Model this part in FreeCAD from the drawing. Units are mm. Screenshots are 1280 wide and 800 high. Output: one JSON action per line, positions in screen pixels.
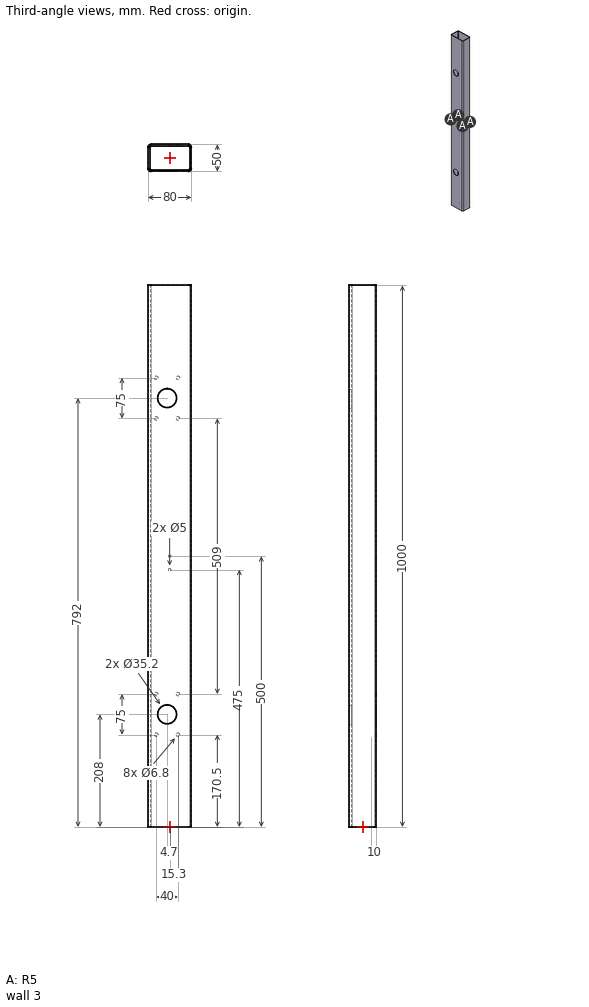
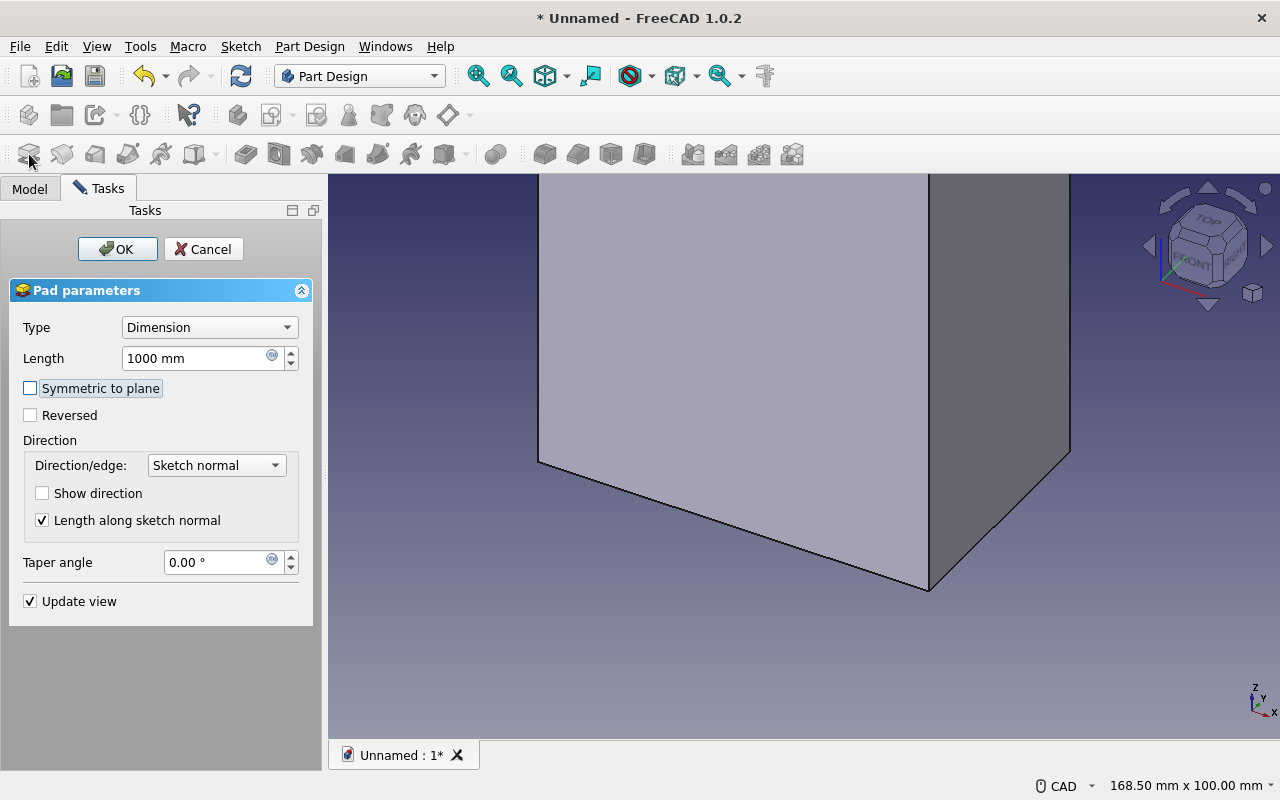
{"action": "left_click", "coordinate": [118, 249]}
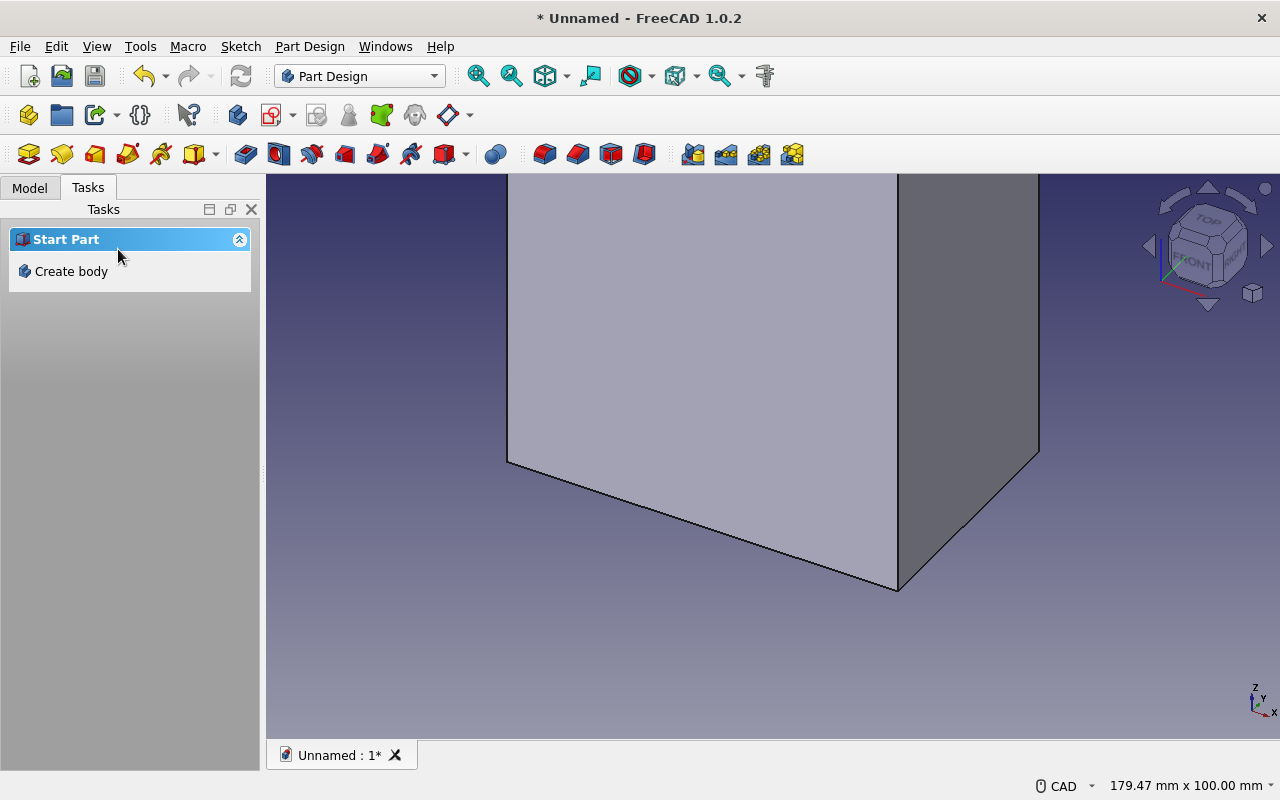
{"action": "left_click", "coordinate": [479, 76]}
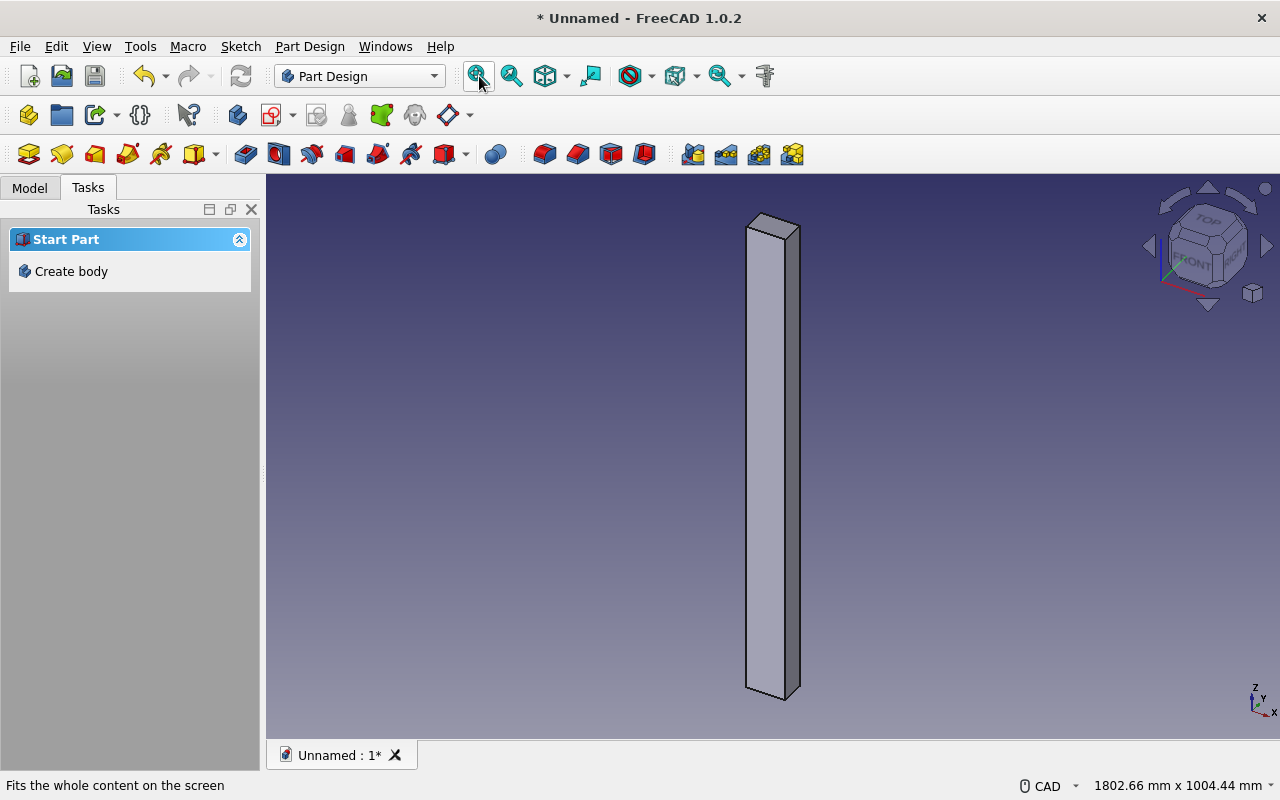
{"action": "left_click", "coordinate": [785, 469]}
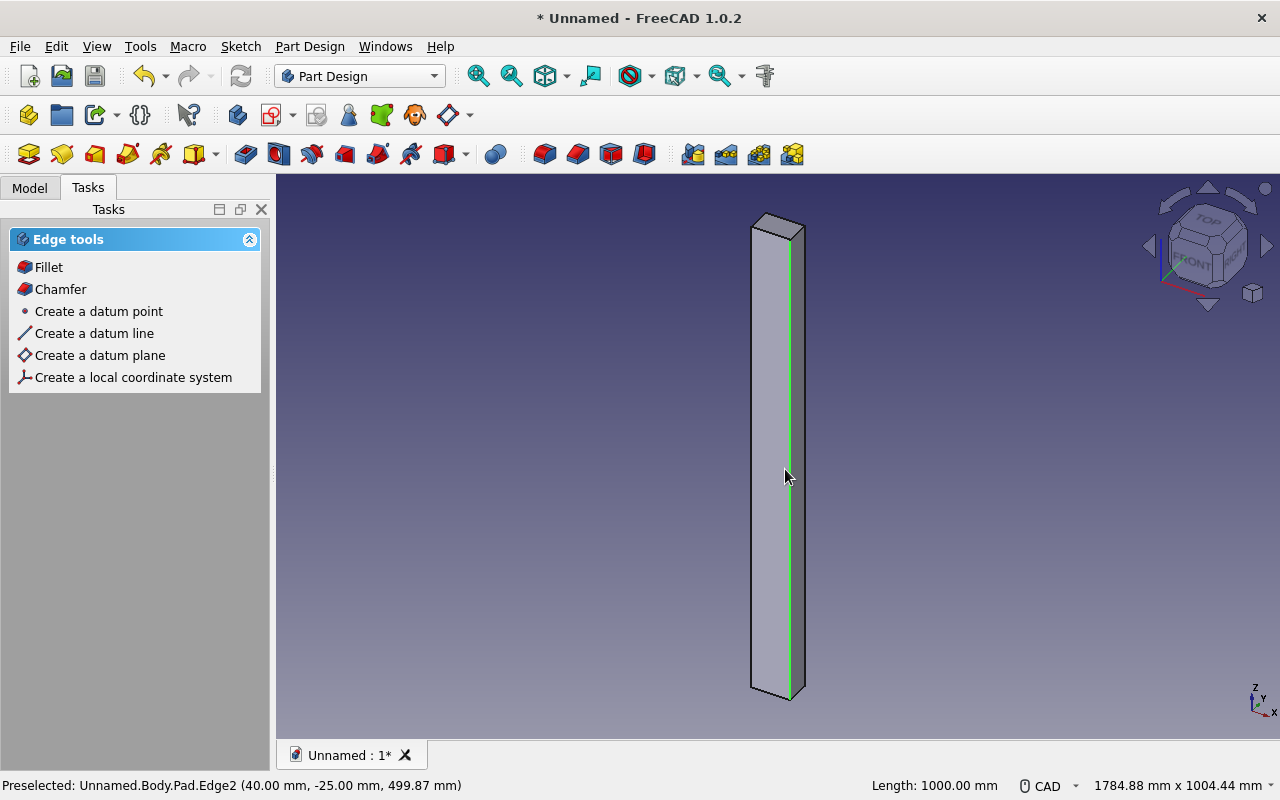
{"action": "key", "text": "0"}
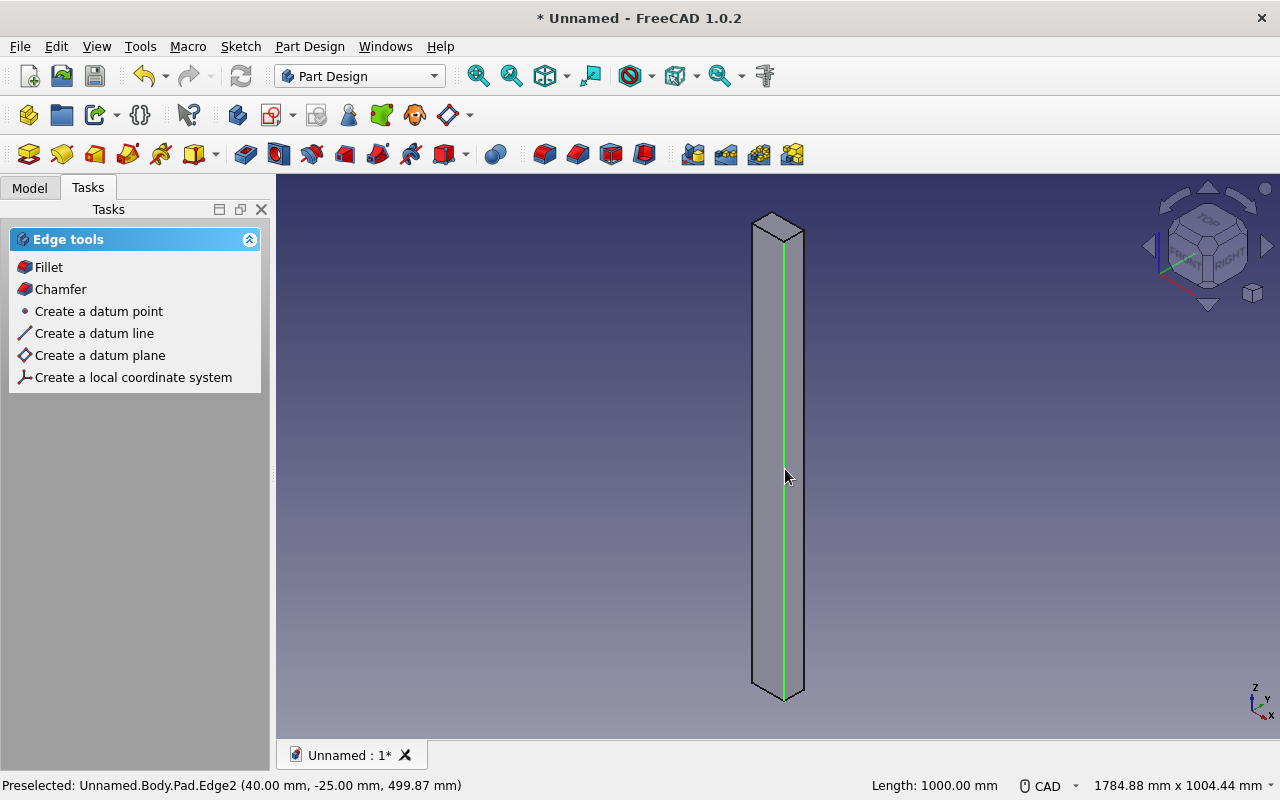
{"action": "key", "text": "2"}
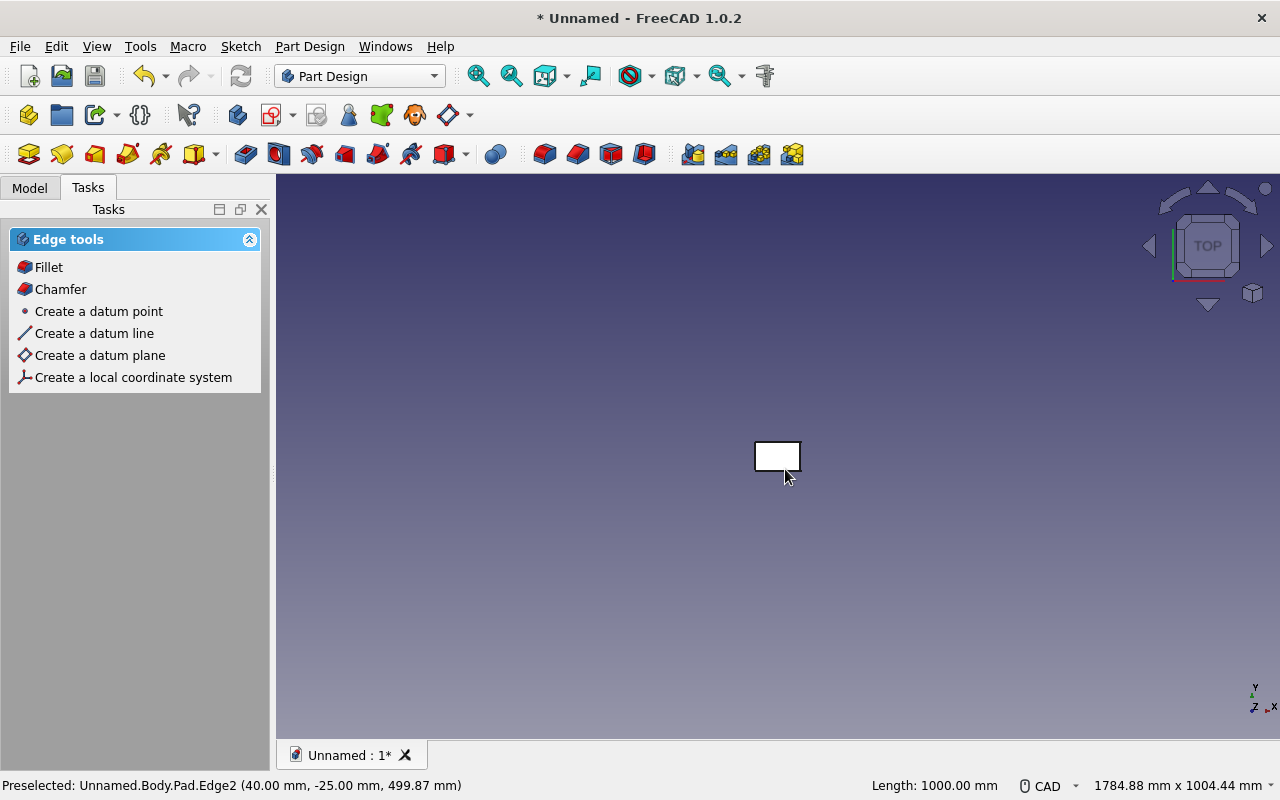
{"action": "left_click", "coordinate": [479, 76]}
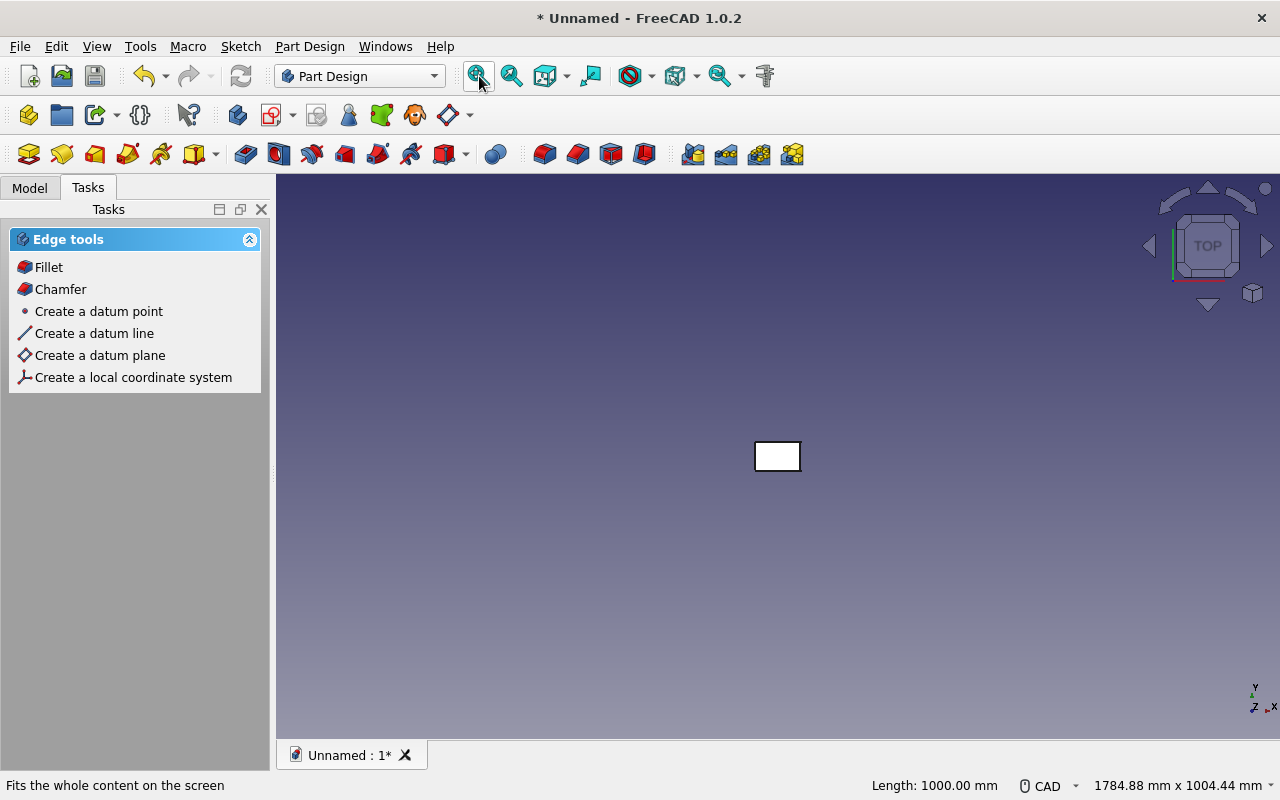
{"action": "key", "text": "1"}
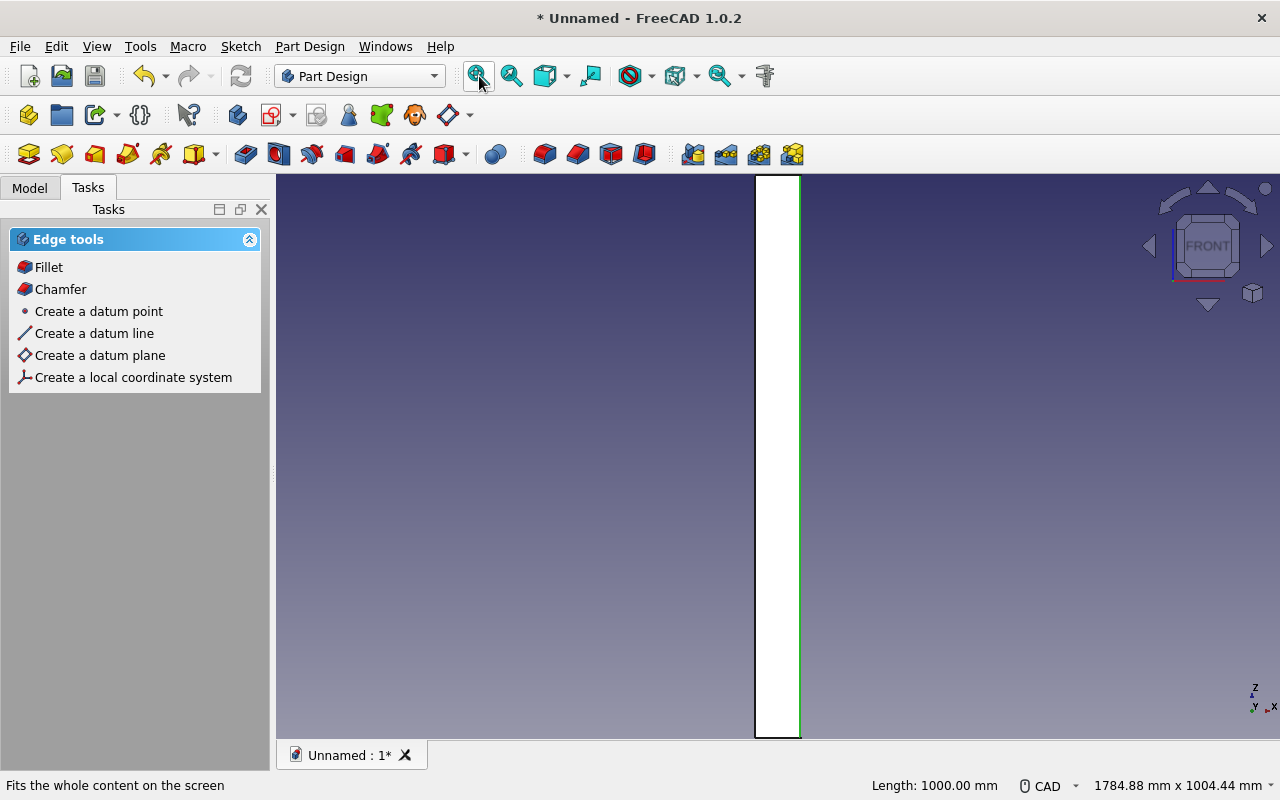
{"action": "left_click", "coordinate": [755, 456], "text": "ctrl"}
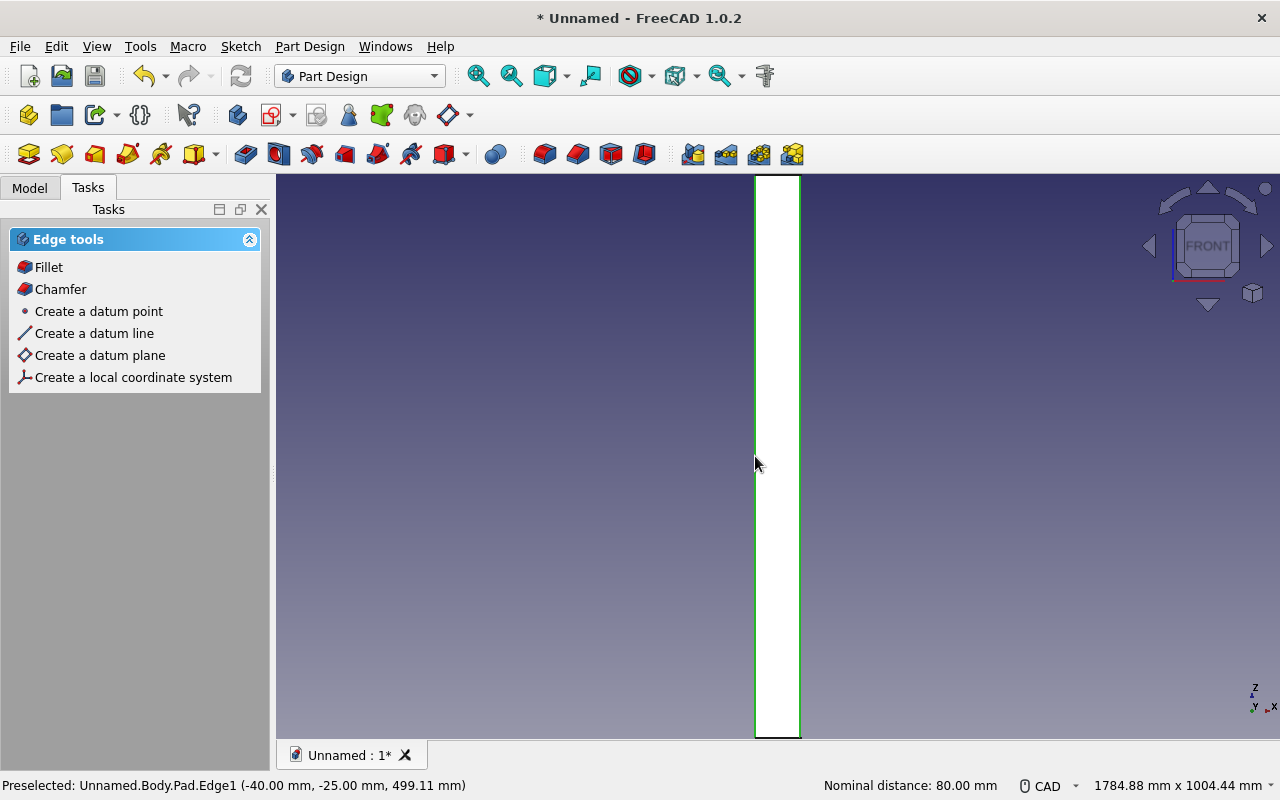
{"action": "key", "text": "3"}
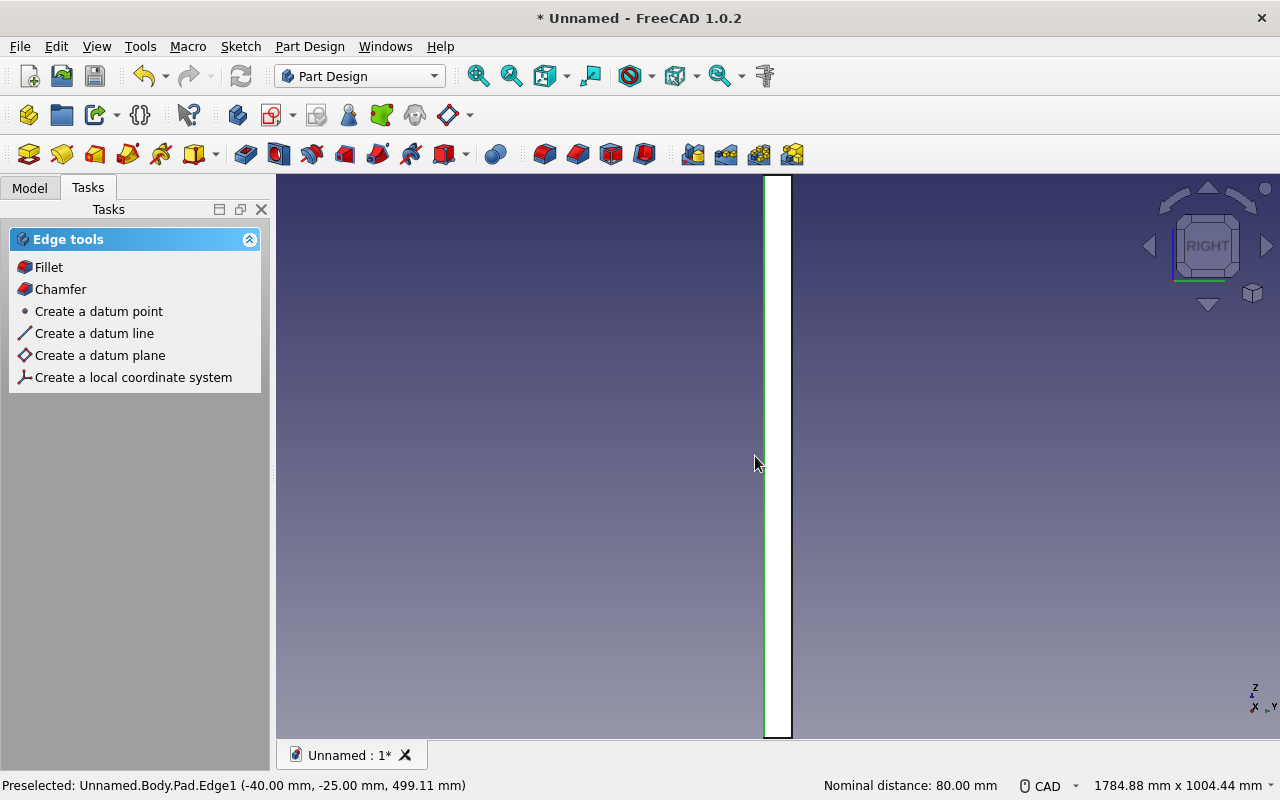
{"action": "left_click", "coordinate": [792, 456], "text": "ctrl"}